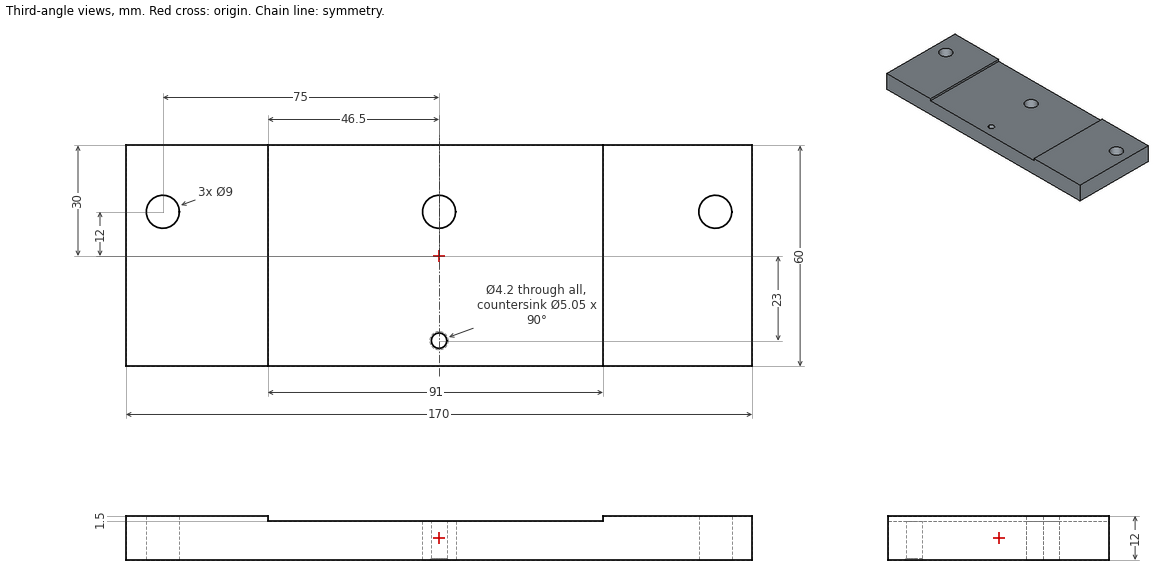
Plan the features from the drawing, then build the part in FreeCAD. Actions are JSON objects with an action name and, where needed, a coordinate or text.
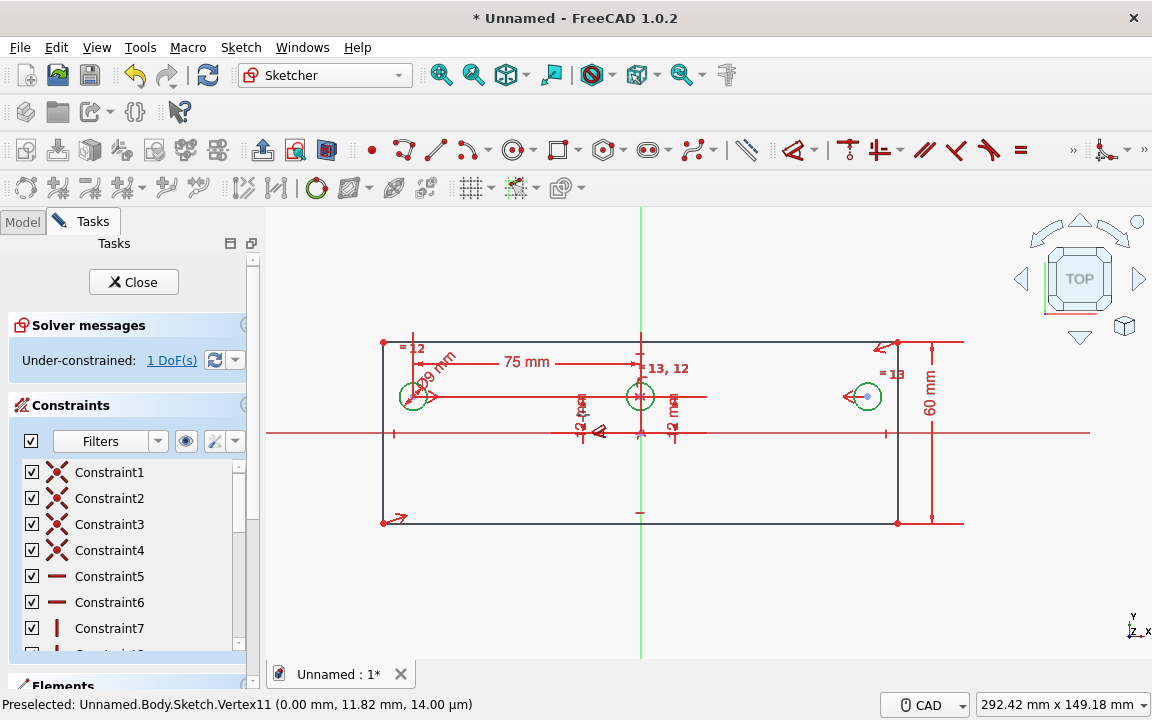
{"action": "left_click", "coordinate": [538, 524]}
{"action": "left_click", "coordinate": [522, 558]}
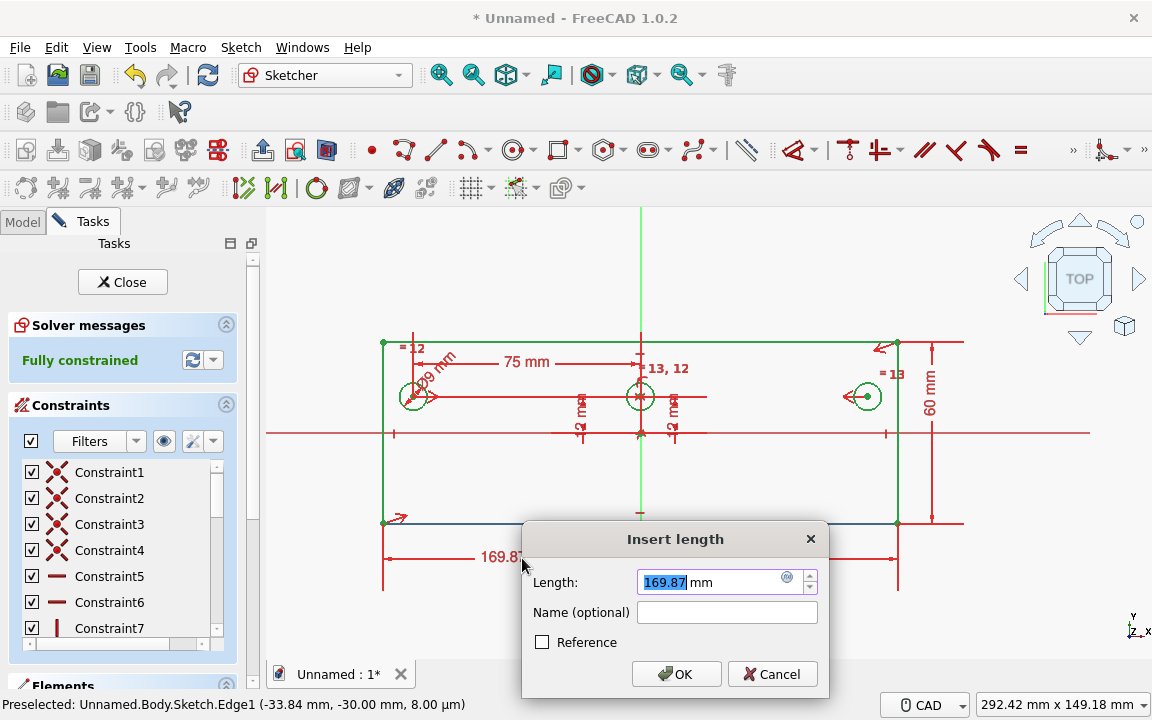
{"action": "type", "text": "170"}
{"action": "key", "text": "Return"}
{"action": "key", "text": "Escape"}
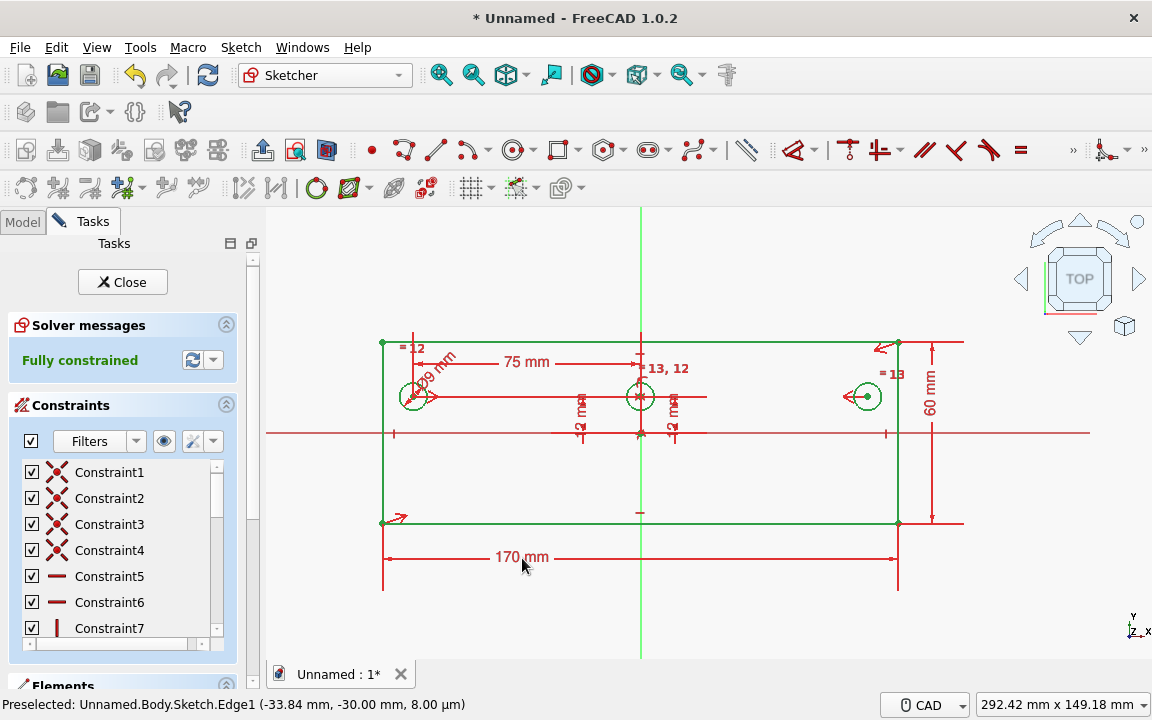
{"action": "left_click", "coordinate": [123, 282]}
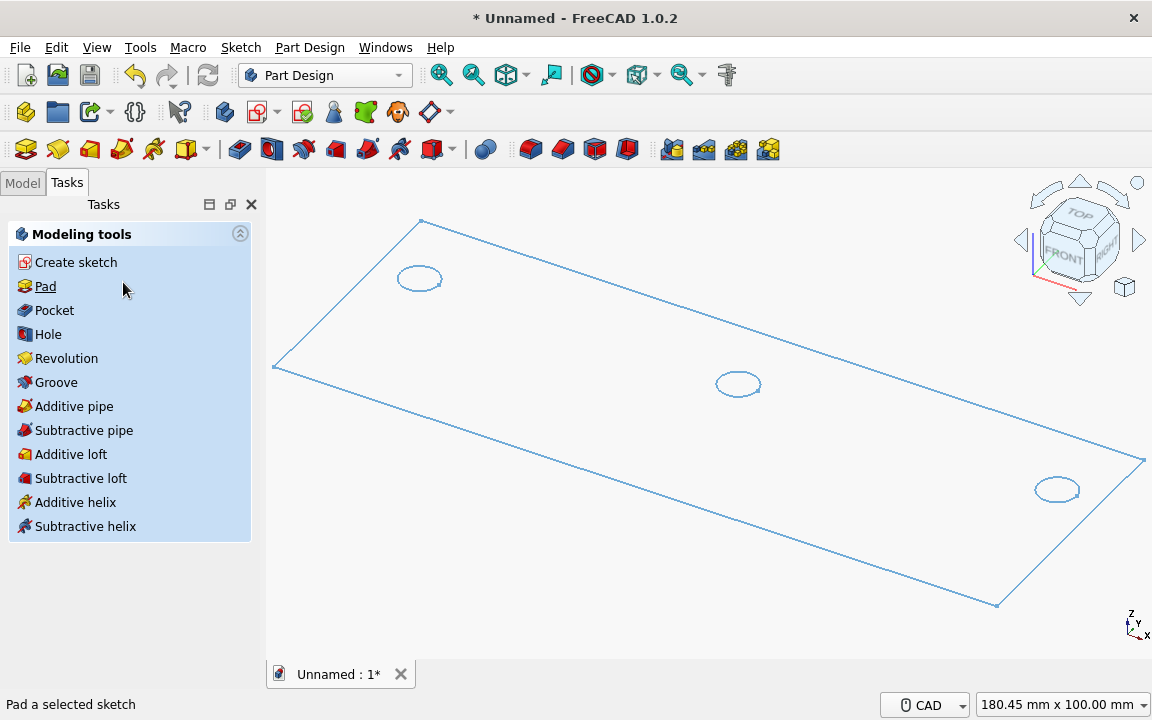
{"action": "left_click", "coordinate": [26, 150]}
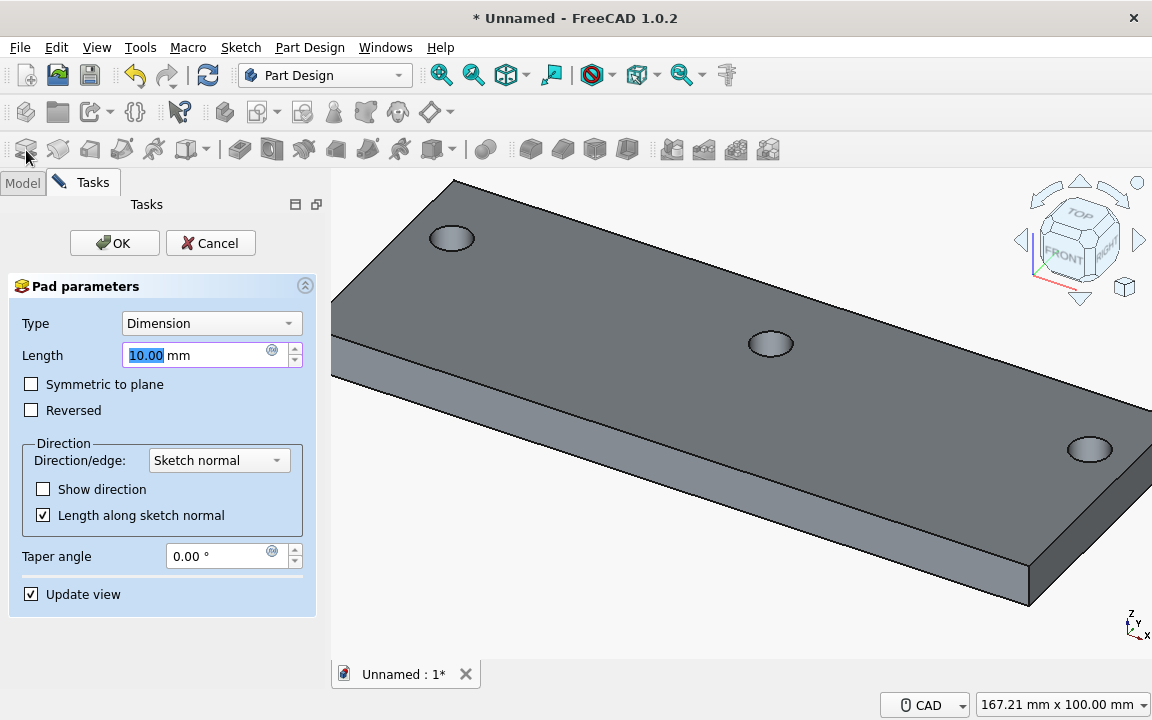
{"action": "type", "text": "12"}
{"action": "key", "text": "Tab"}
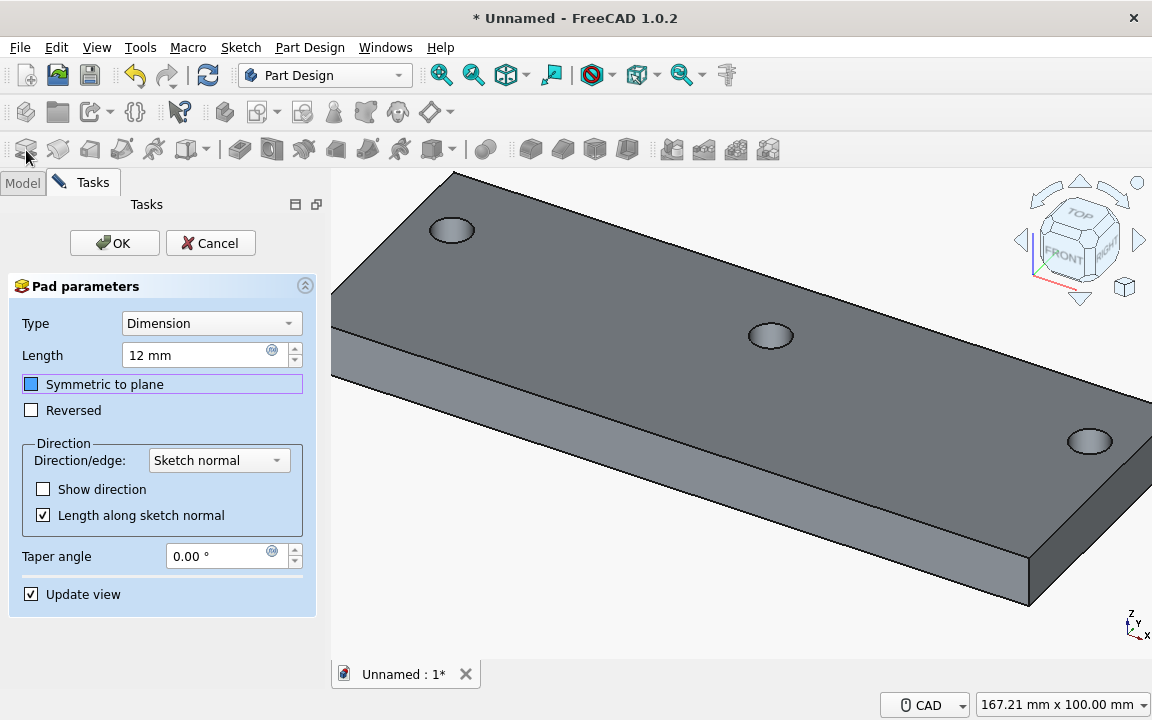
{"action": "left_click", "coordinate": [30, 384]}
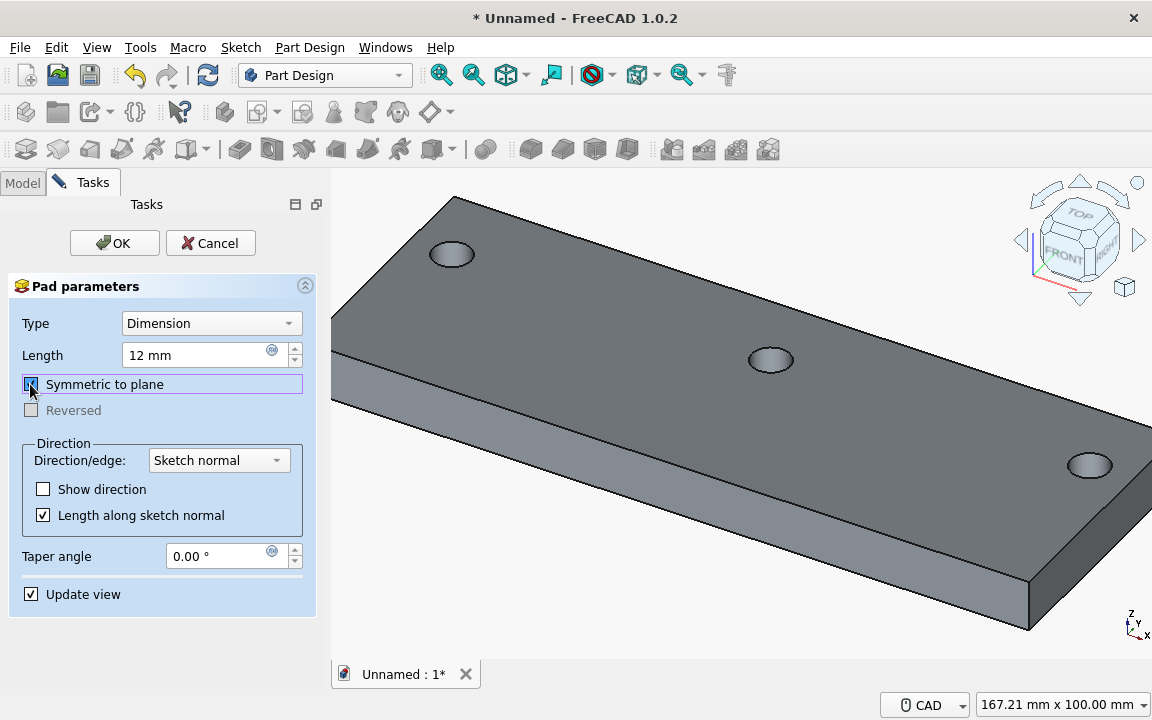
{"action": "left_click", "coordinate": [115, 243]}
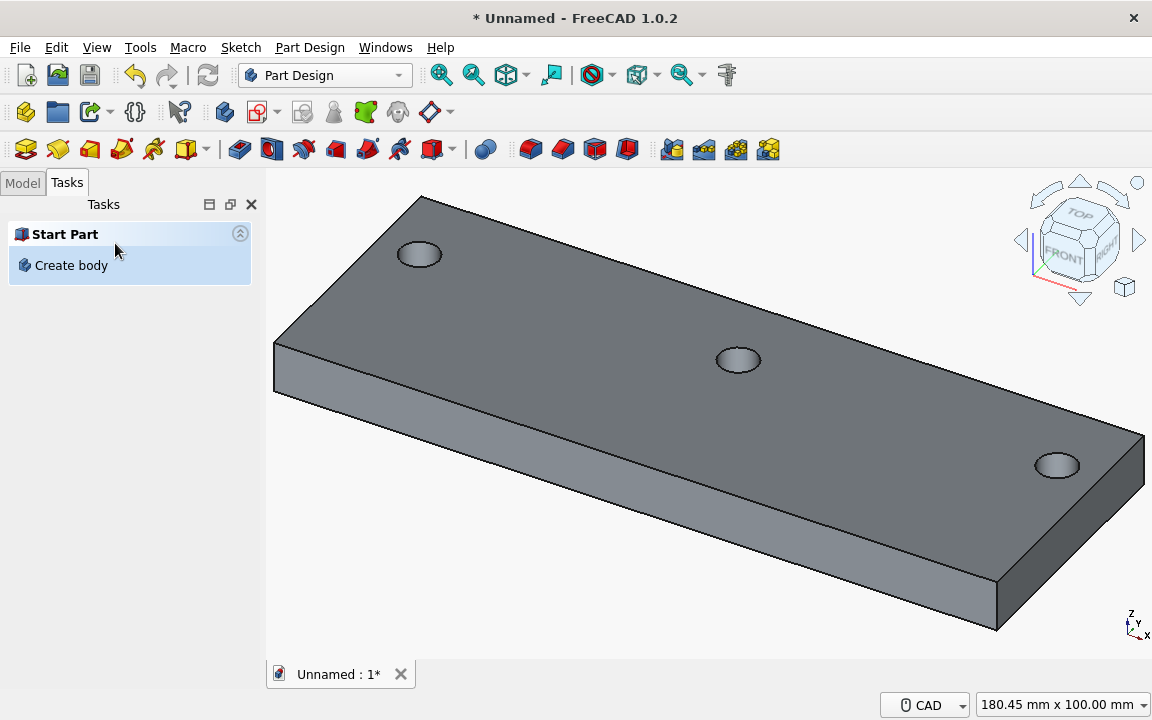
{"action": "left_click", "coordinate": [502, 320]}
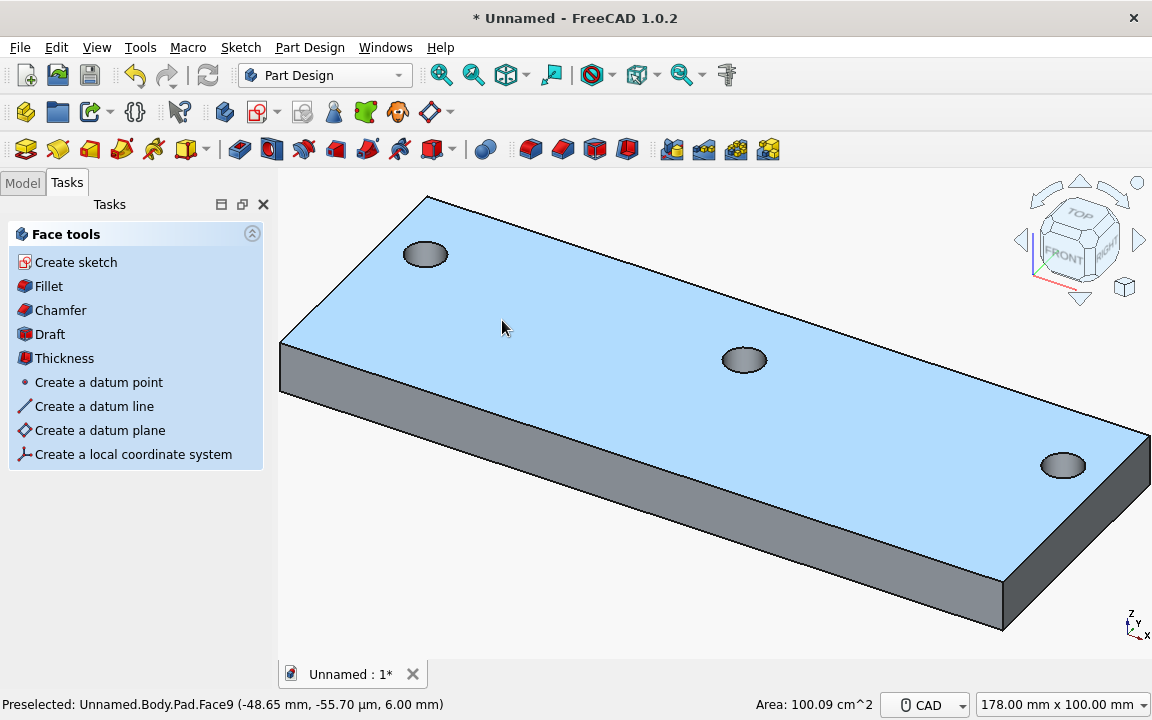
{"action": "left_click", "coordinate": [258, 112]}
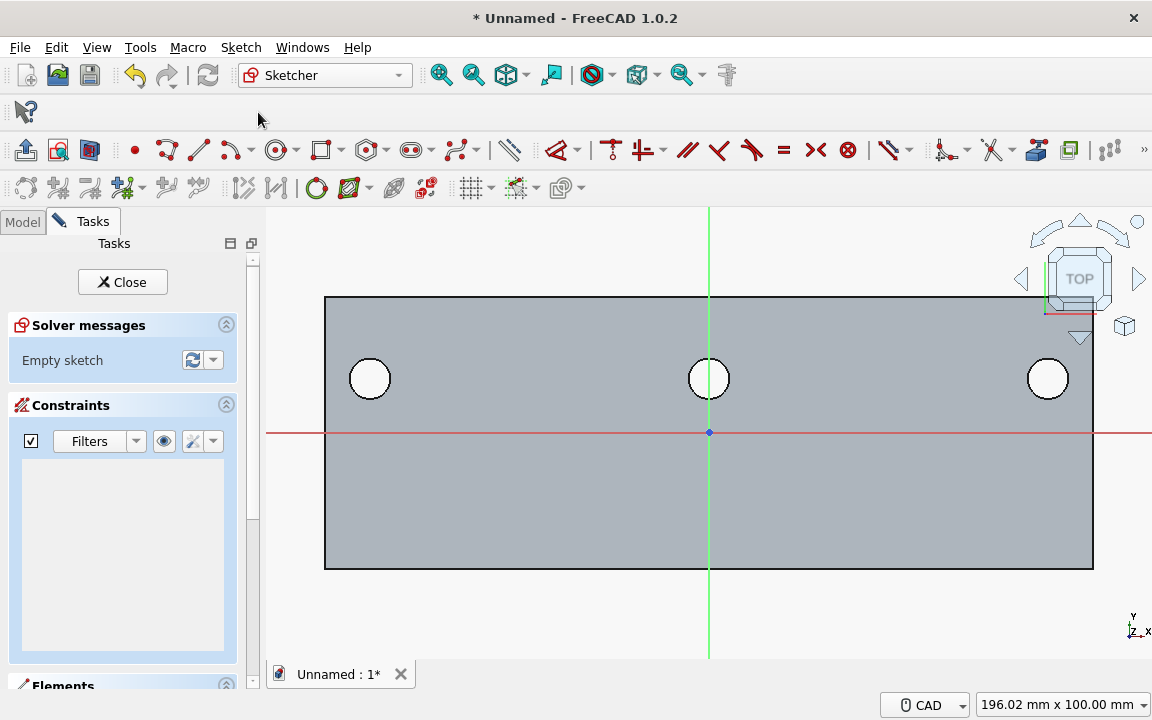
{"action": "key", "text": "g r"}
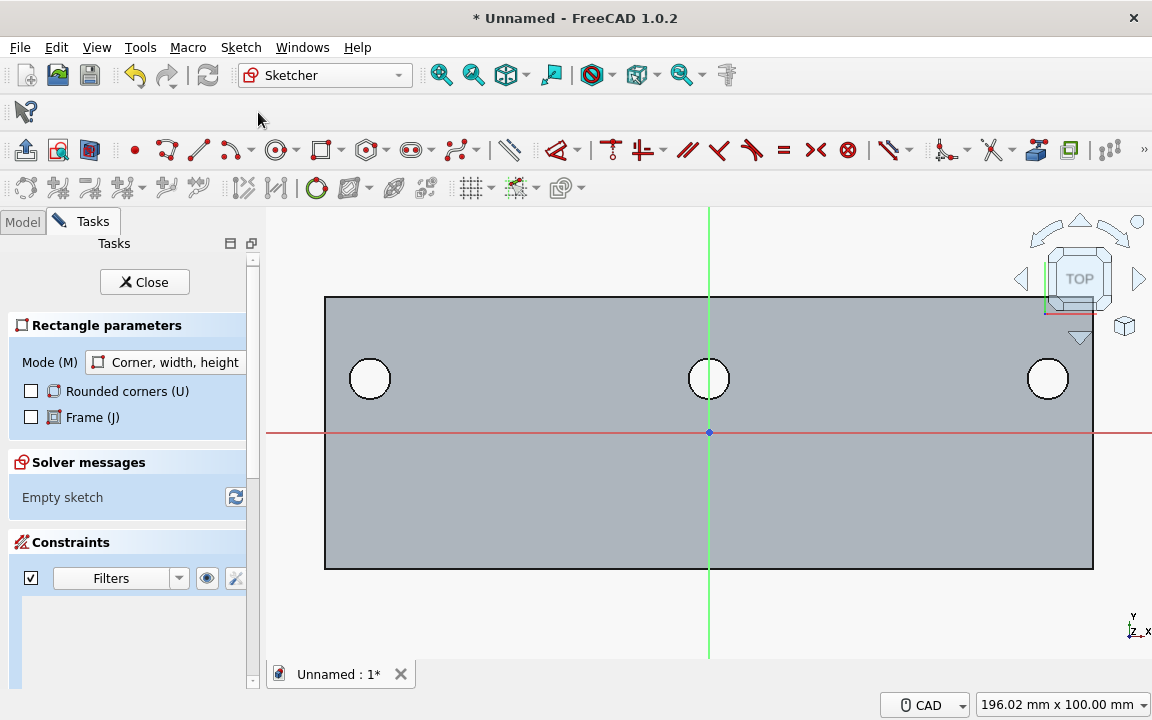
{"action": "left_click", "coordinate": [499, 297]}
{"action": "left_click", "coordinate": [910, 569]}
{"action": "key", "text": "Escape"}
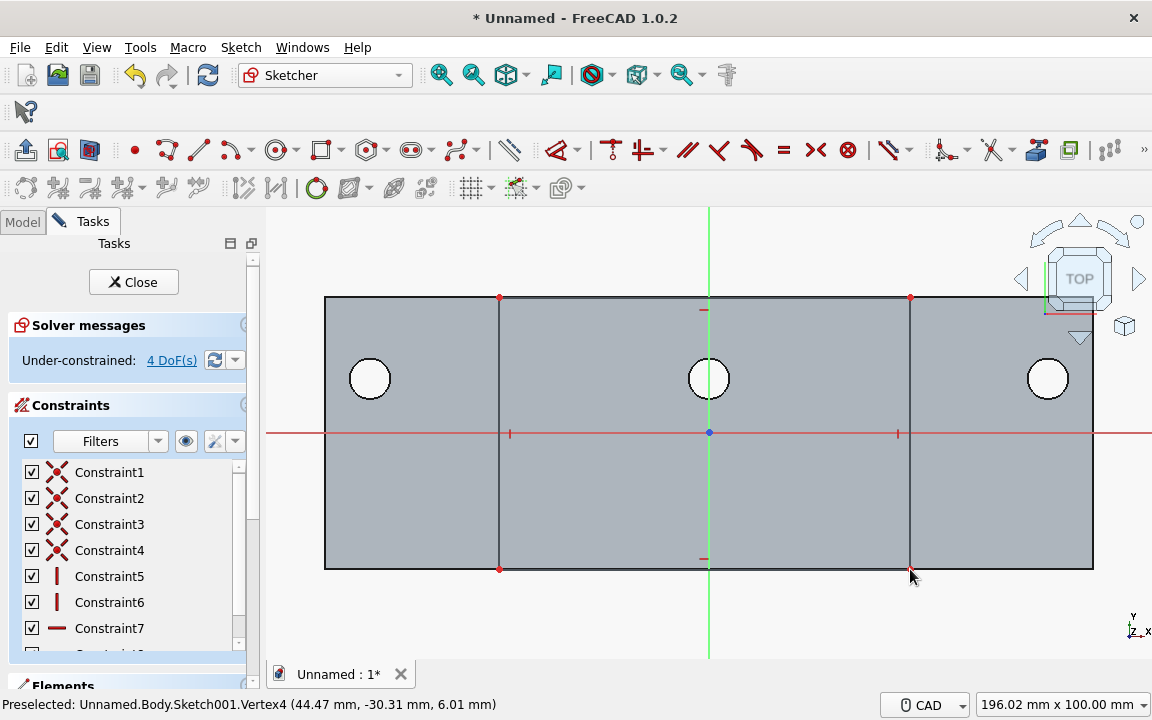
{"action": "left_click", "coordinate": [556, 150]}